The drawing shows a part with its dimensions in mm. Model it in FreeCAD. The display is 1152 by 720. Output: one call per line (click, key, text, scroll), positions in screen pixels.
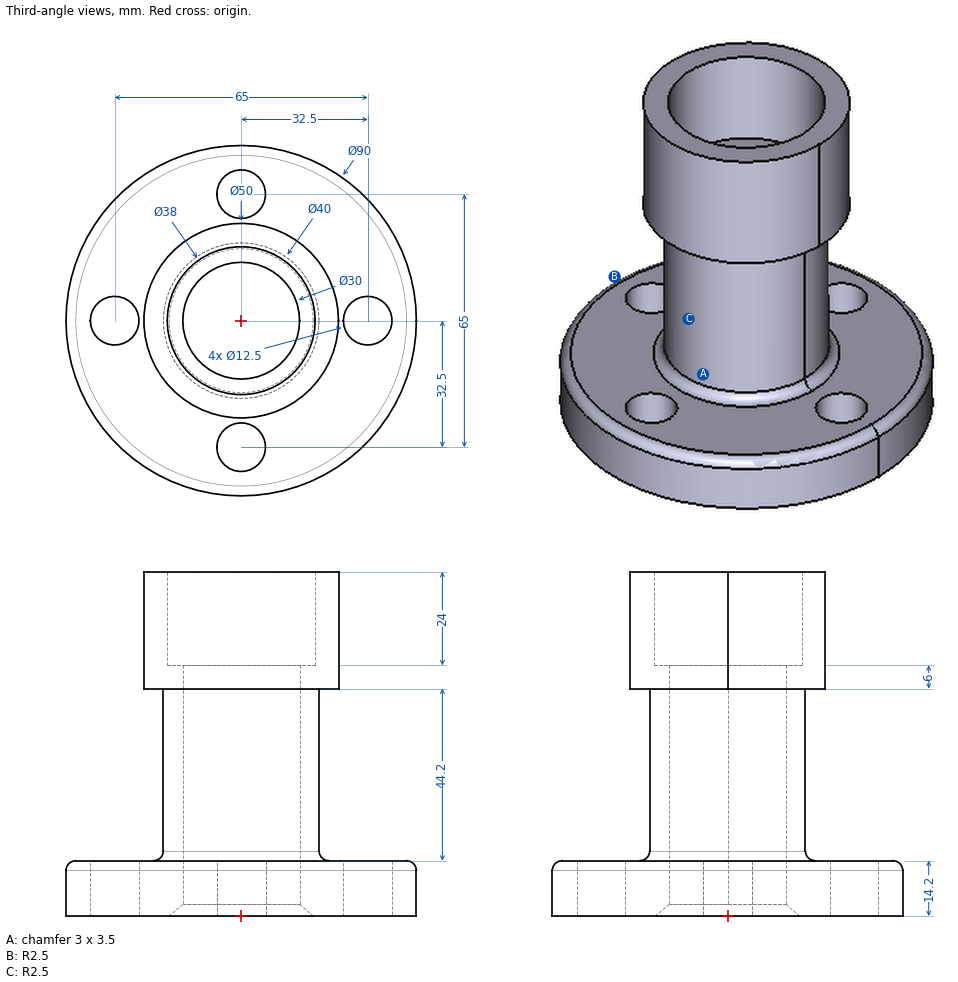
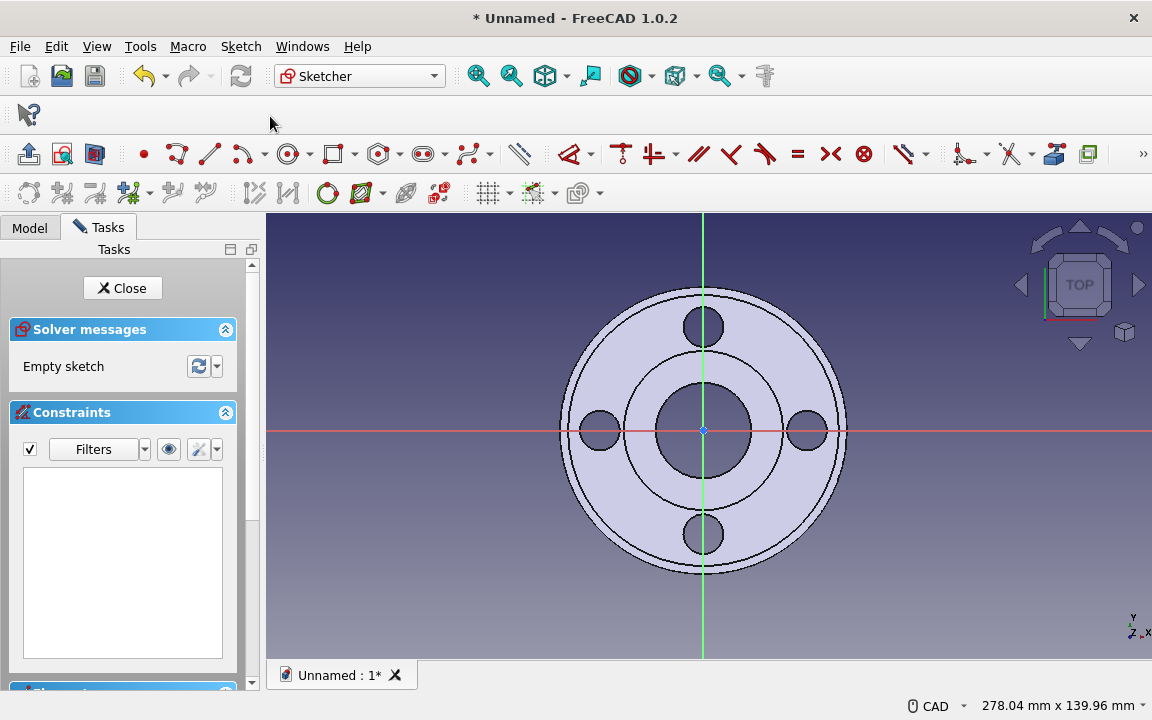
scroll(780, 424, up, 3)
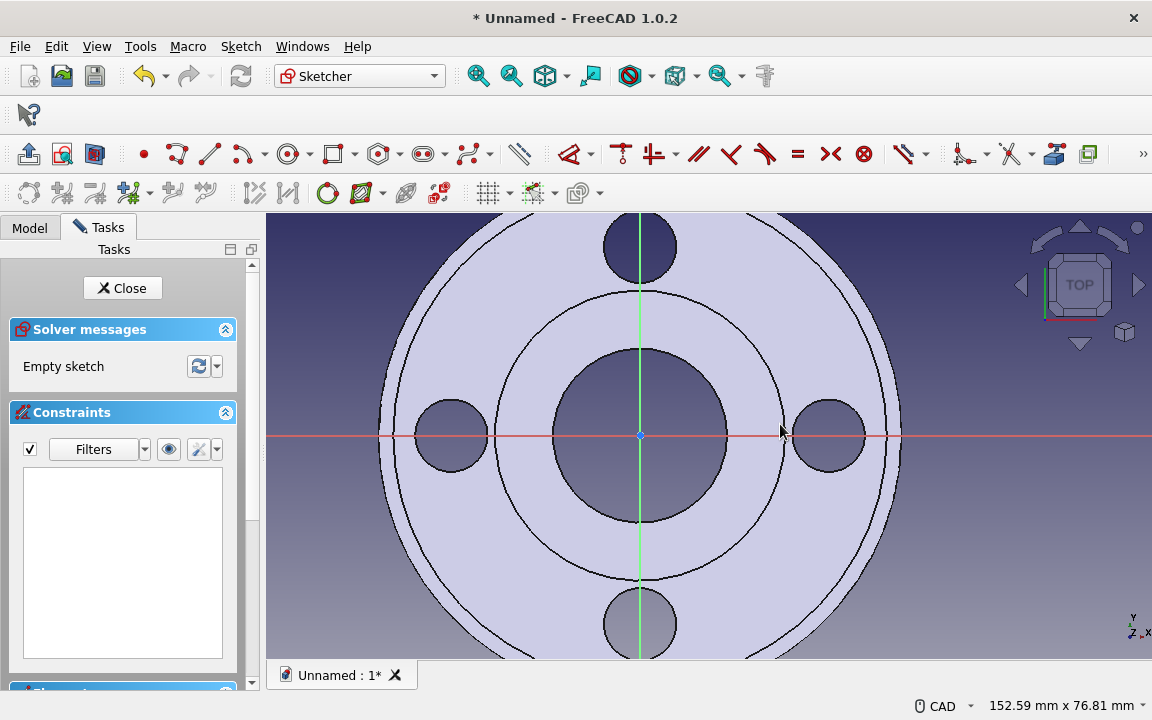
click(288, 154)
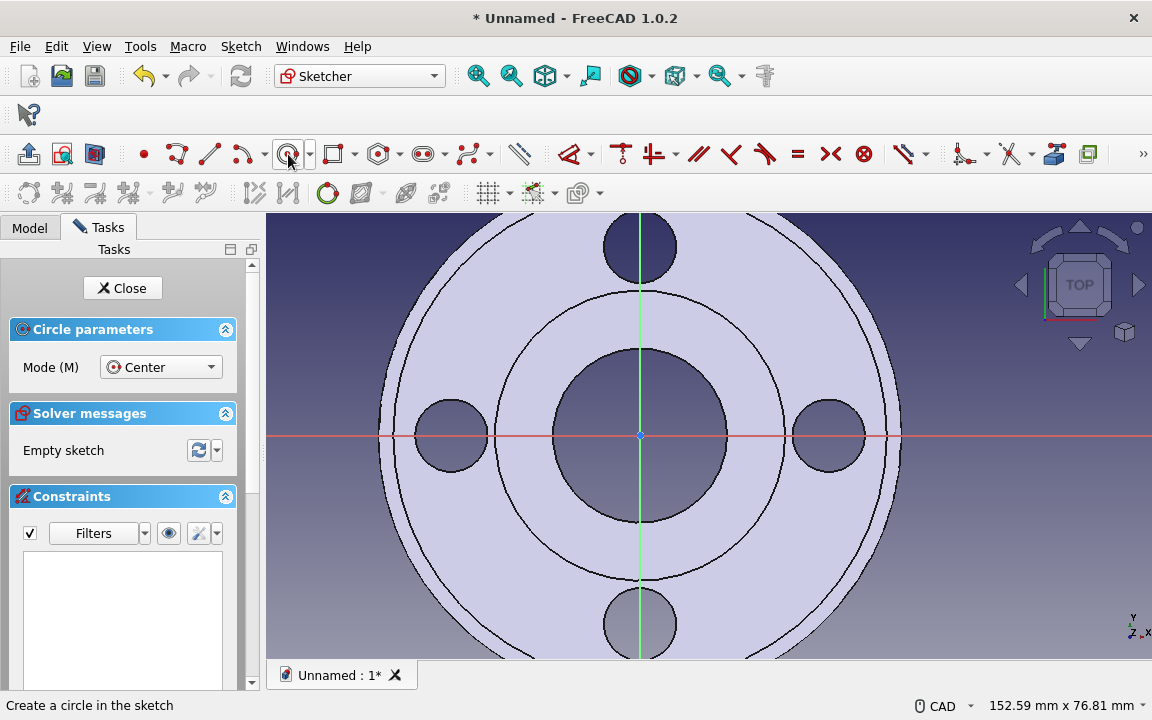
click(640, 436)
click(743, 333)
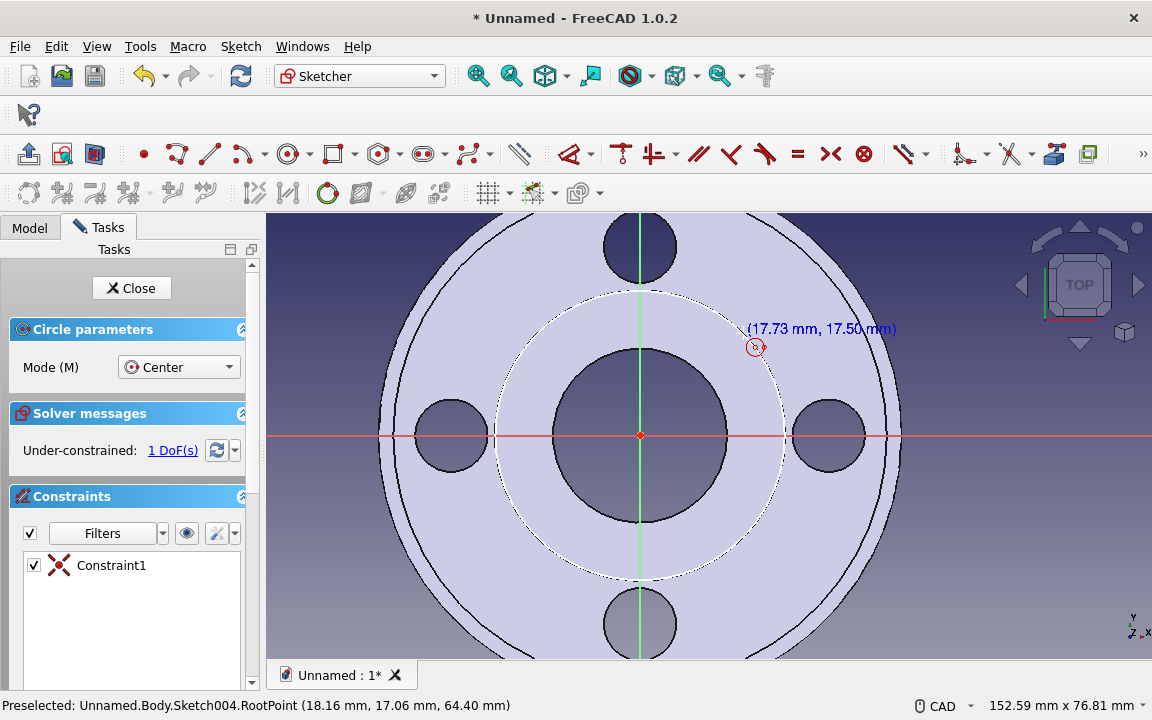
click(640, 436)
click(718, 358)
key(Escape)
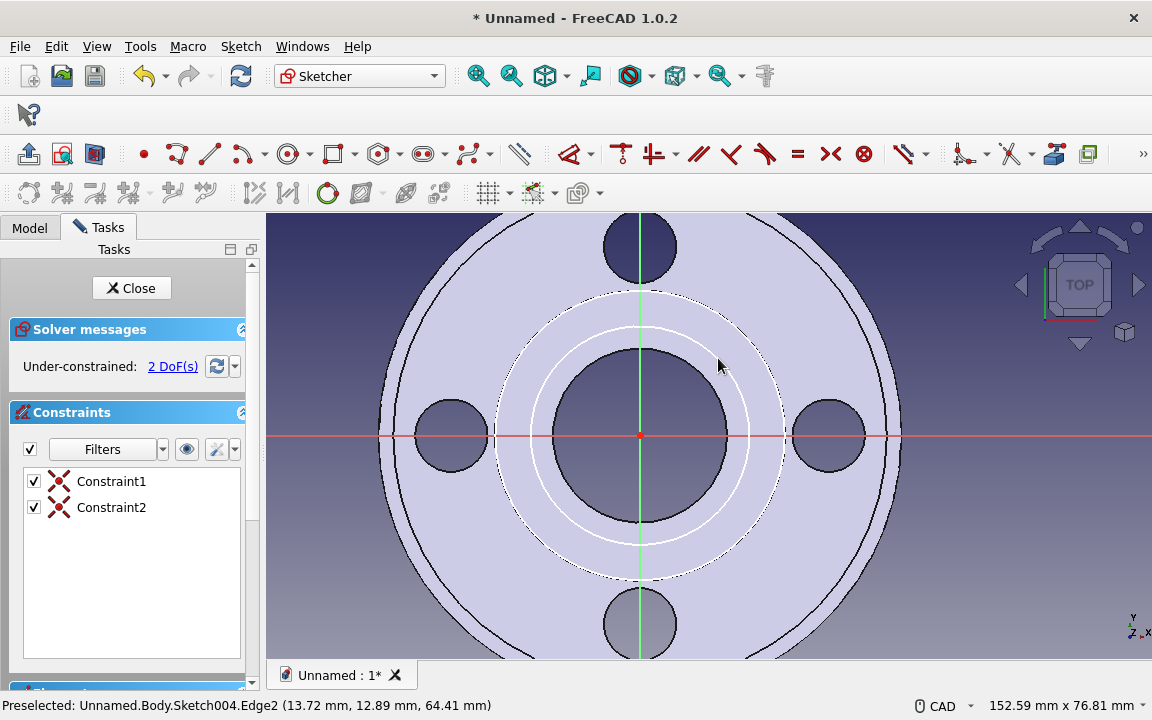
click(568, 154)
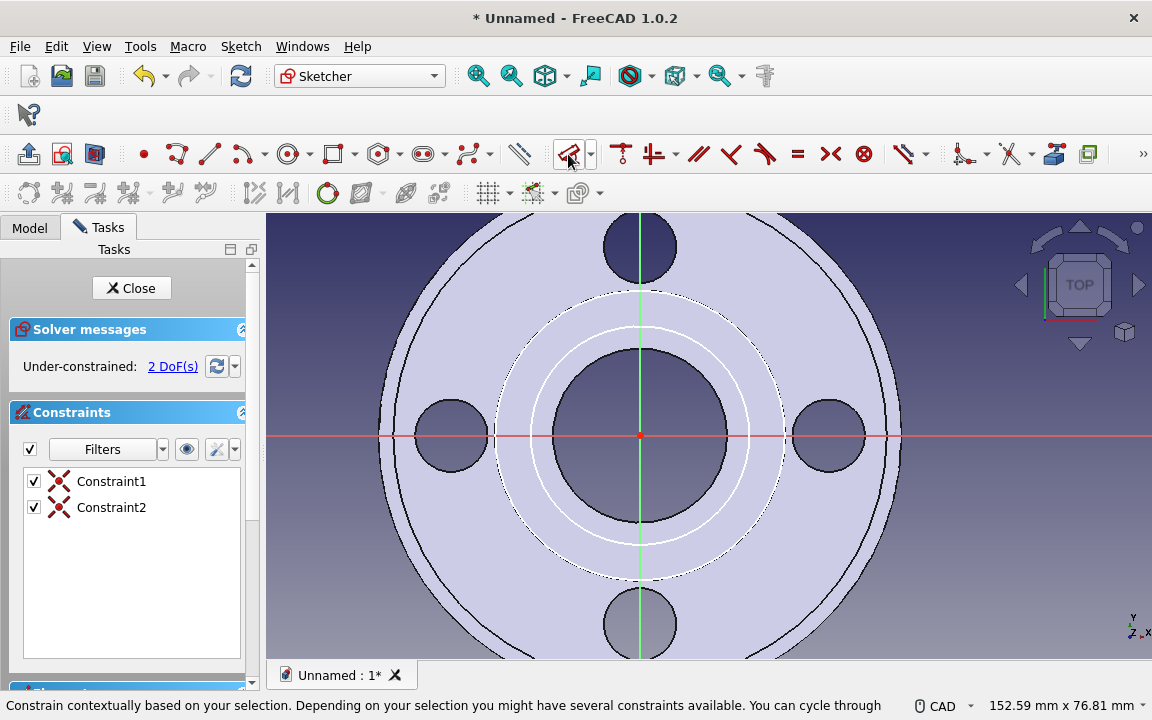
click(742, 333)
click(765, 310)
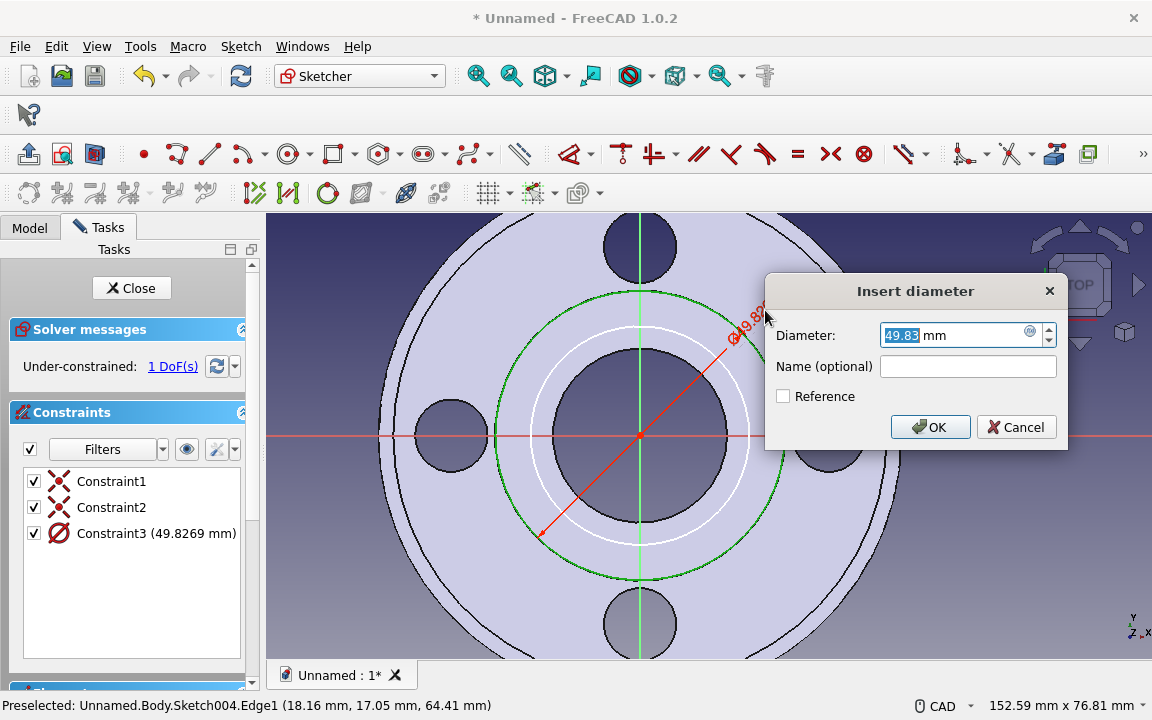
text(50)
key(Return)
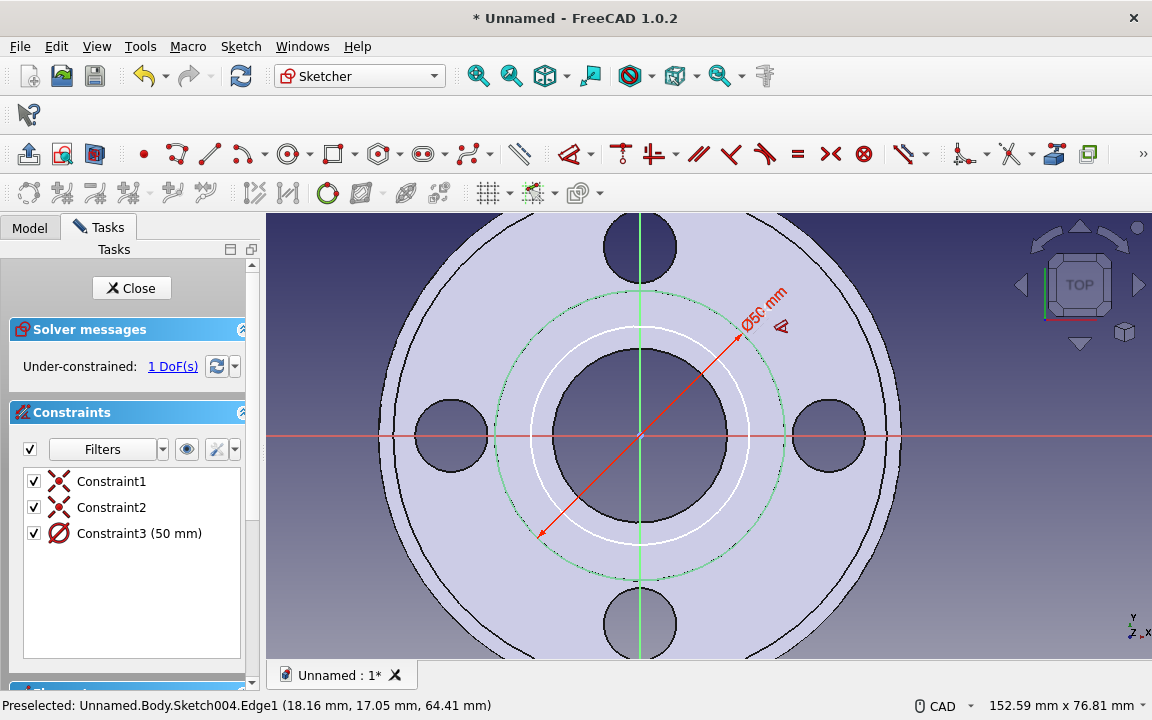
click(717, 358)
click(797, 389)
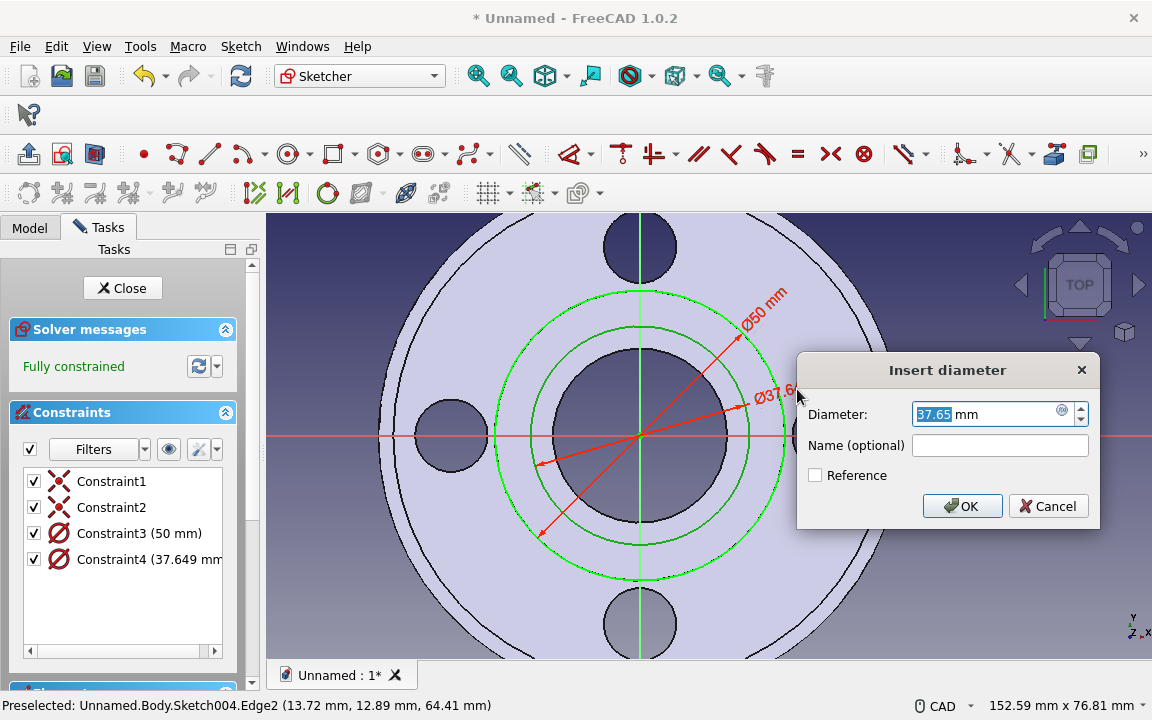
text(38)
key(Return)
key(Escape)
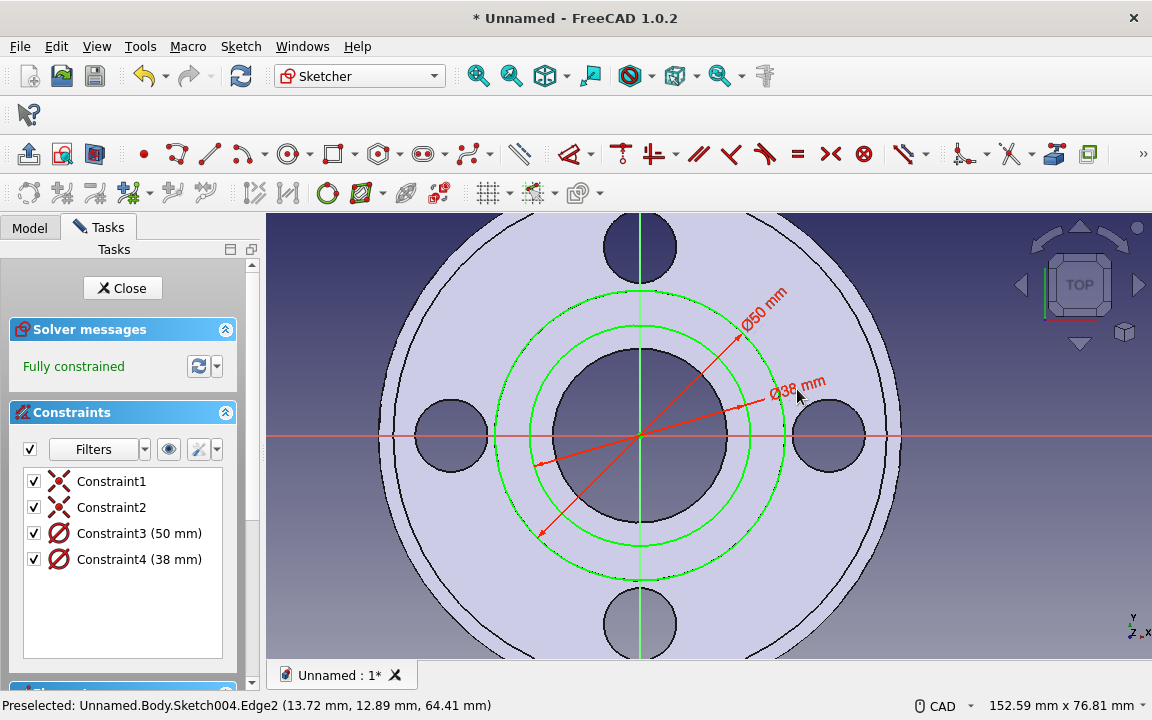
click(123, 288)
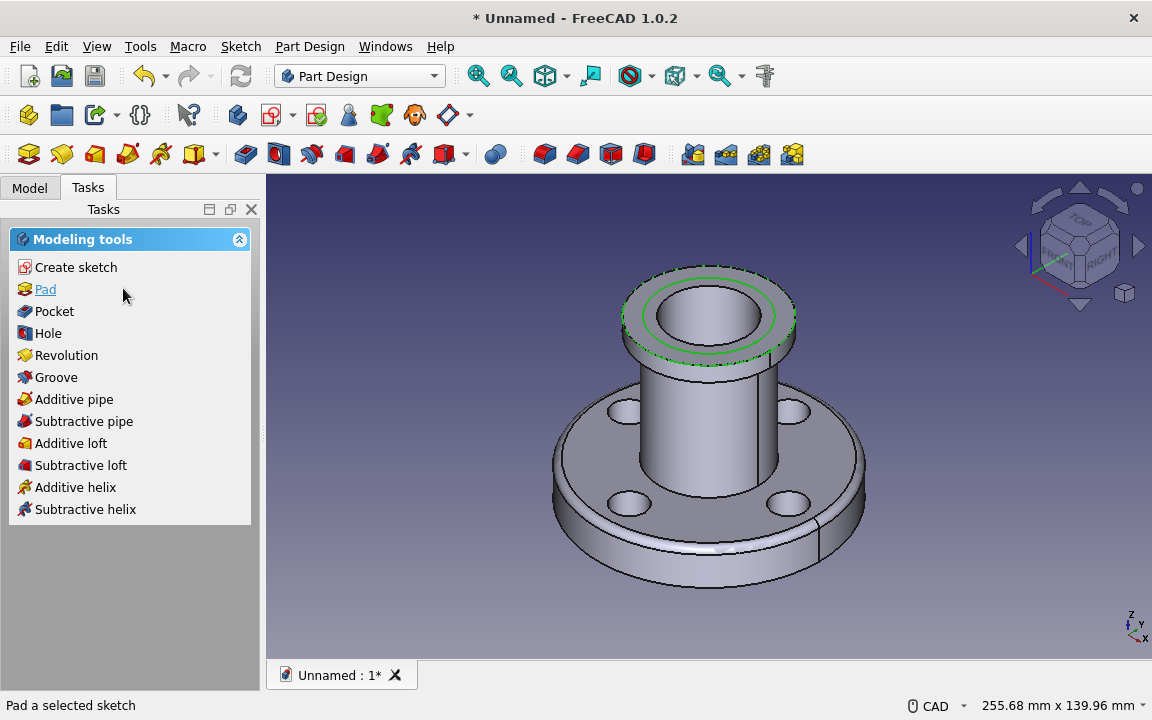
click(29, 154)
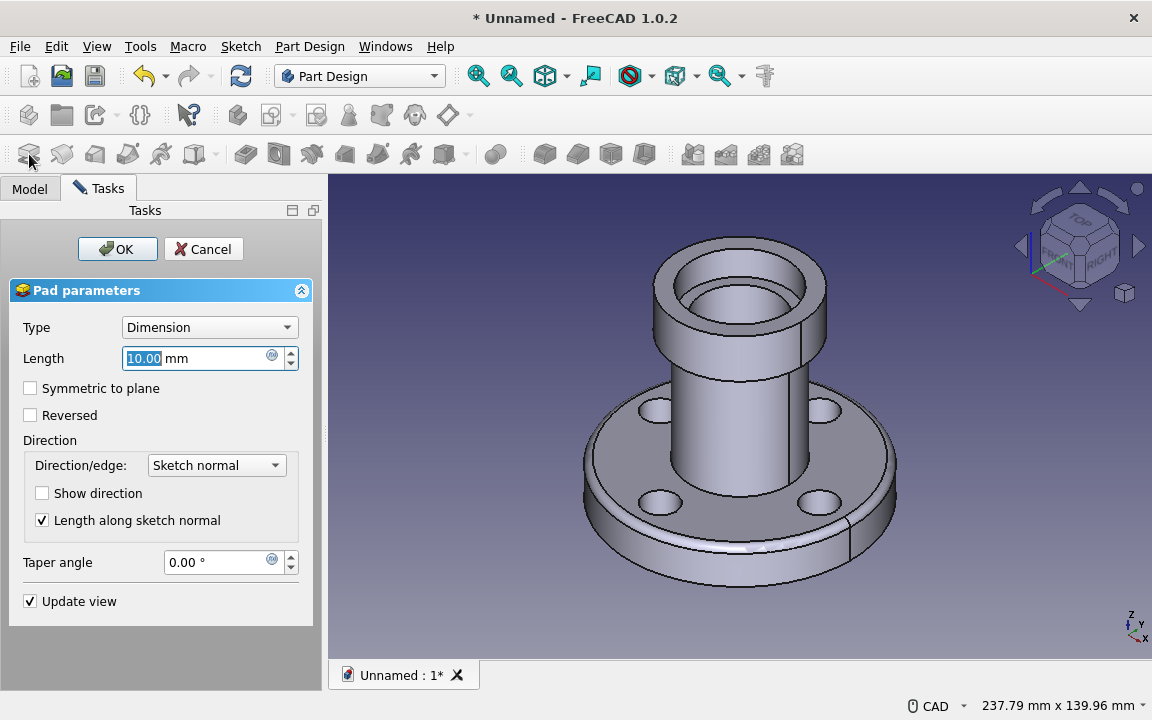
text(24)
key(Tab)